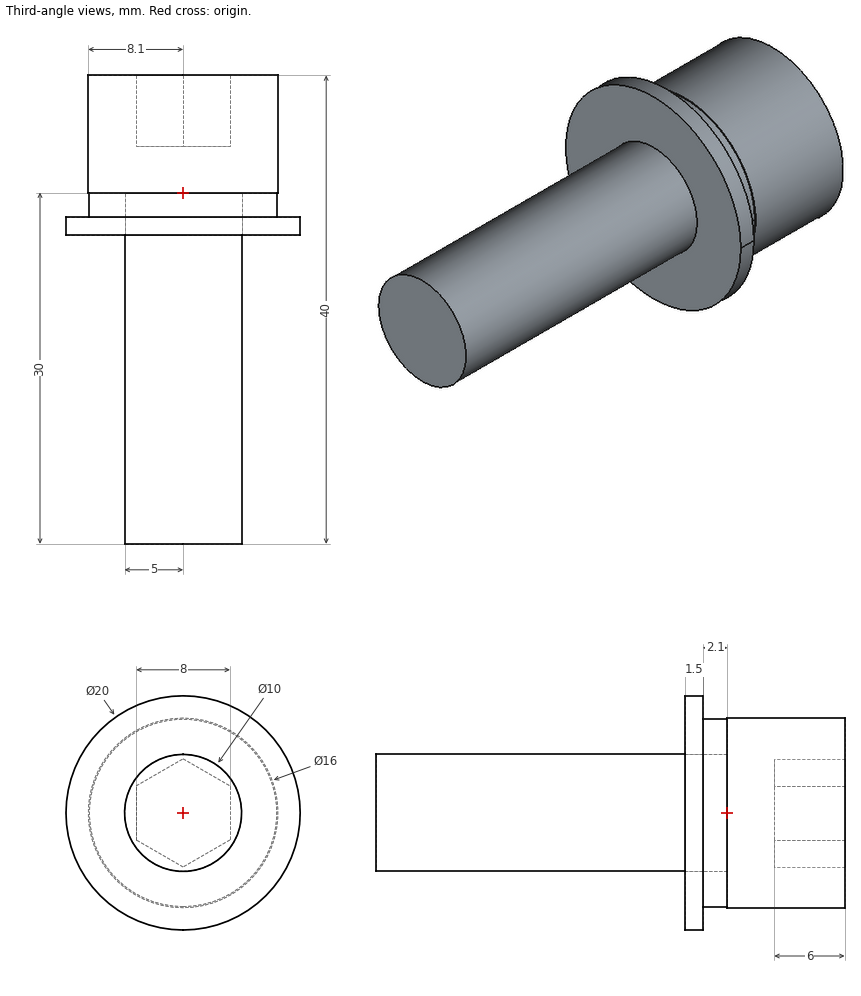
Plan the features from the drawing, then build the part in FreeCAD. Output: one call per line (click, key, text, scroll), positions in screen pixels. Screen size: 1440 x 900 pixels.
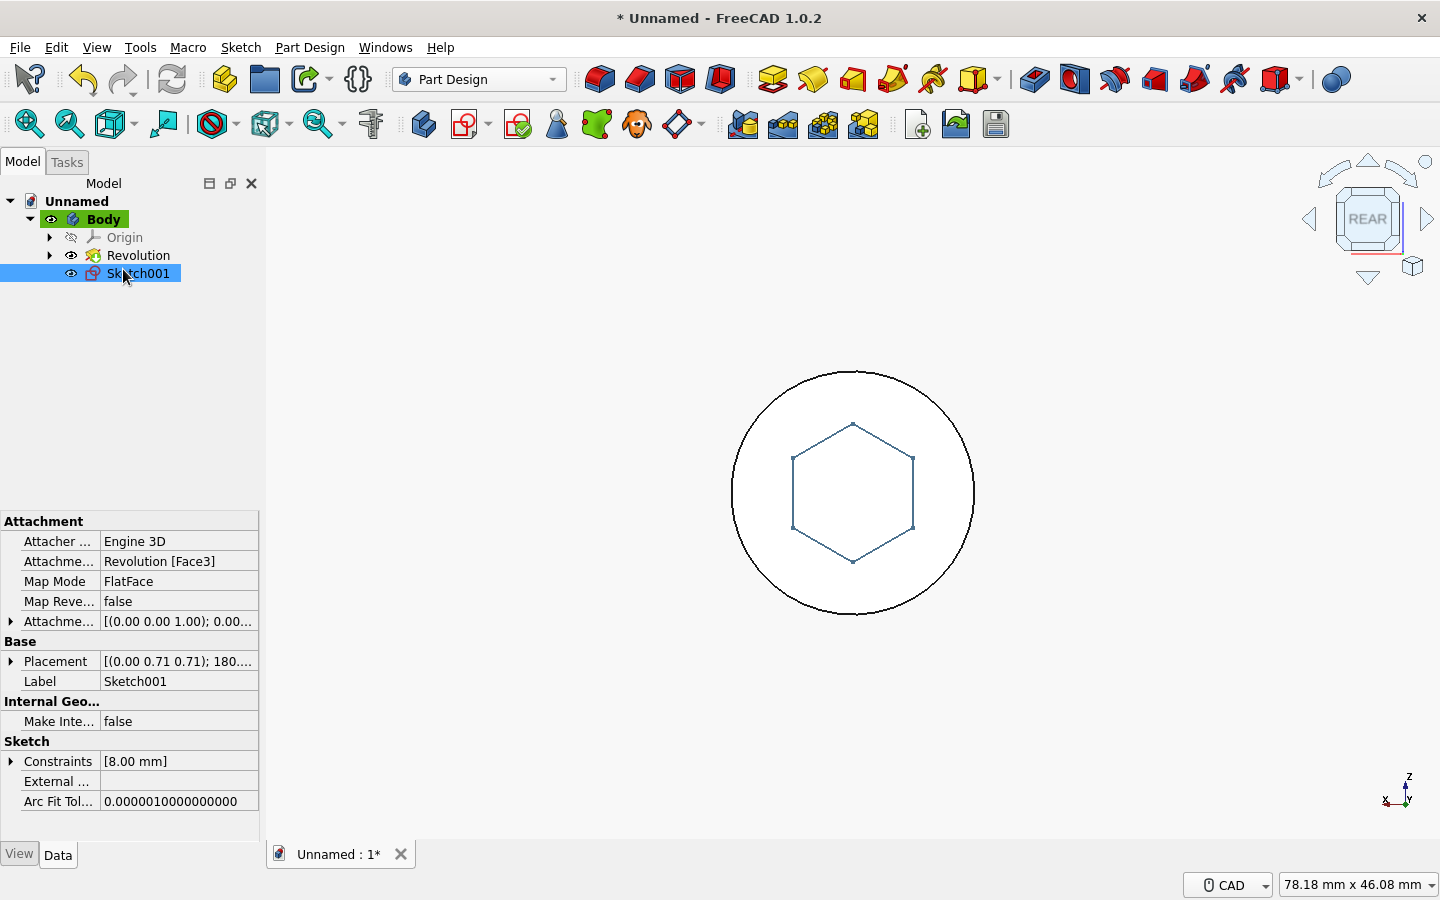
click(1036, 80)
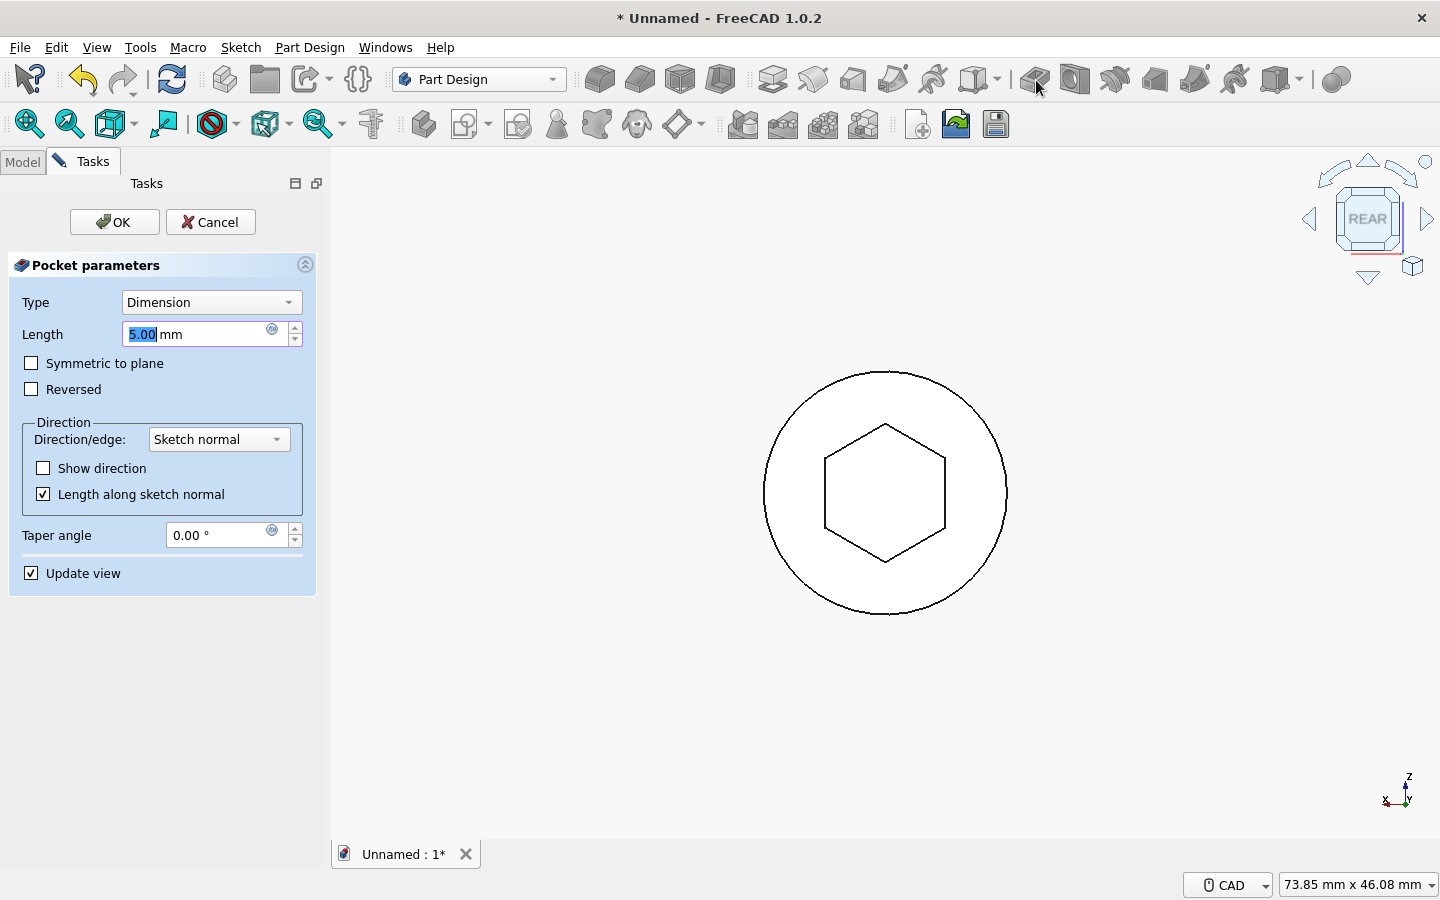
text(6)
key(Tab)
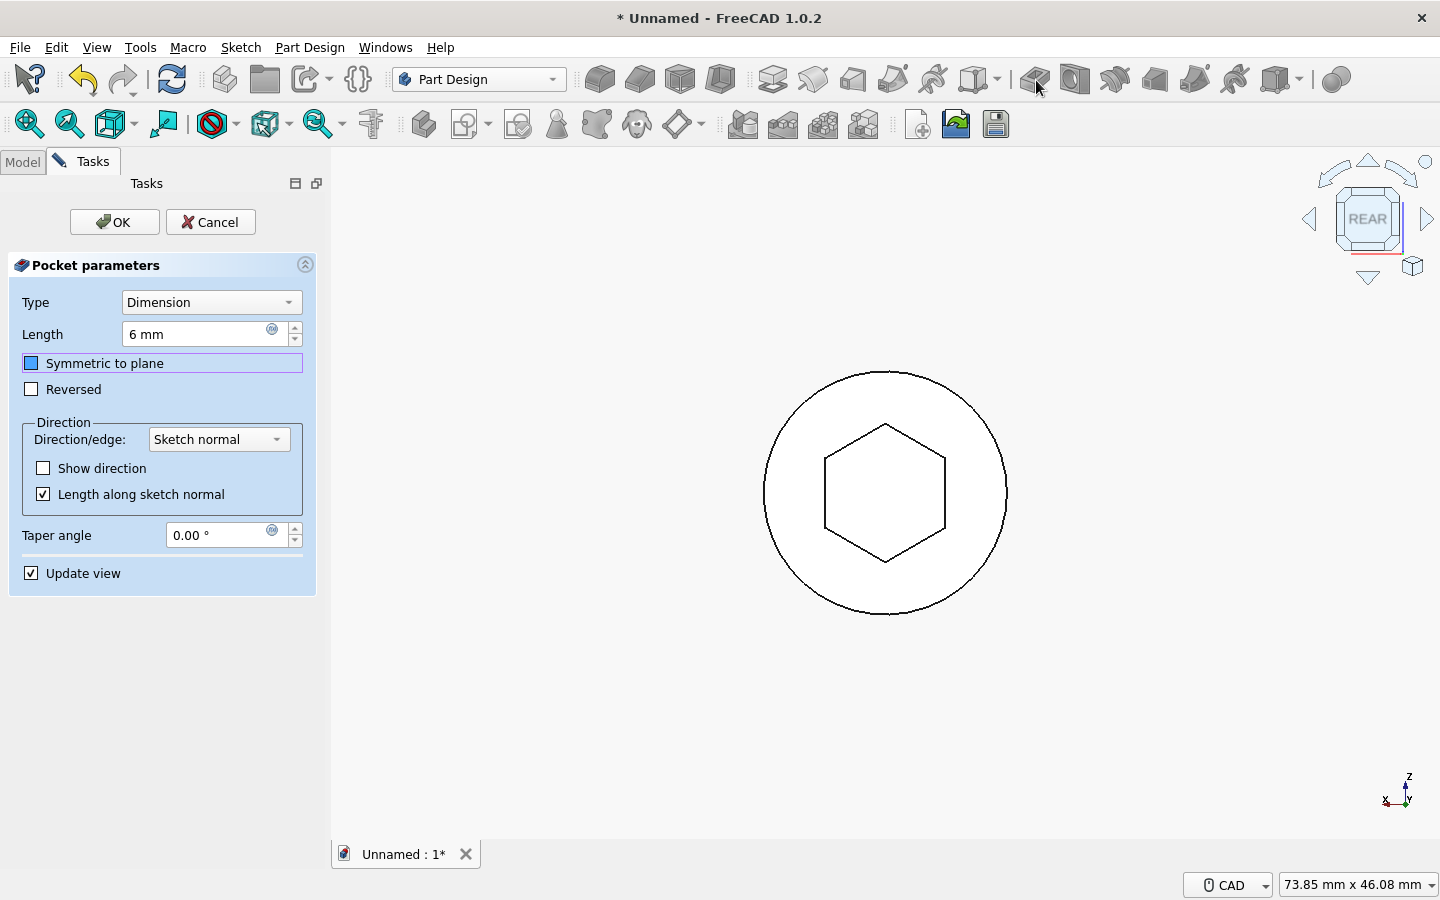
click(115, 222)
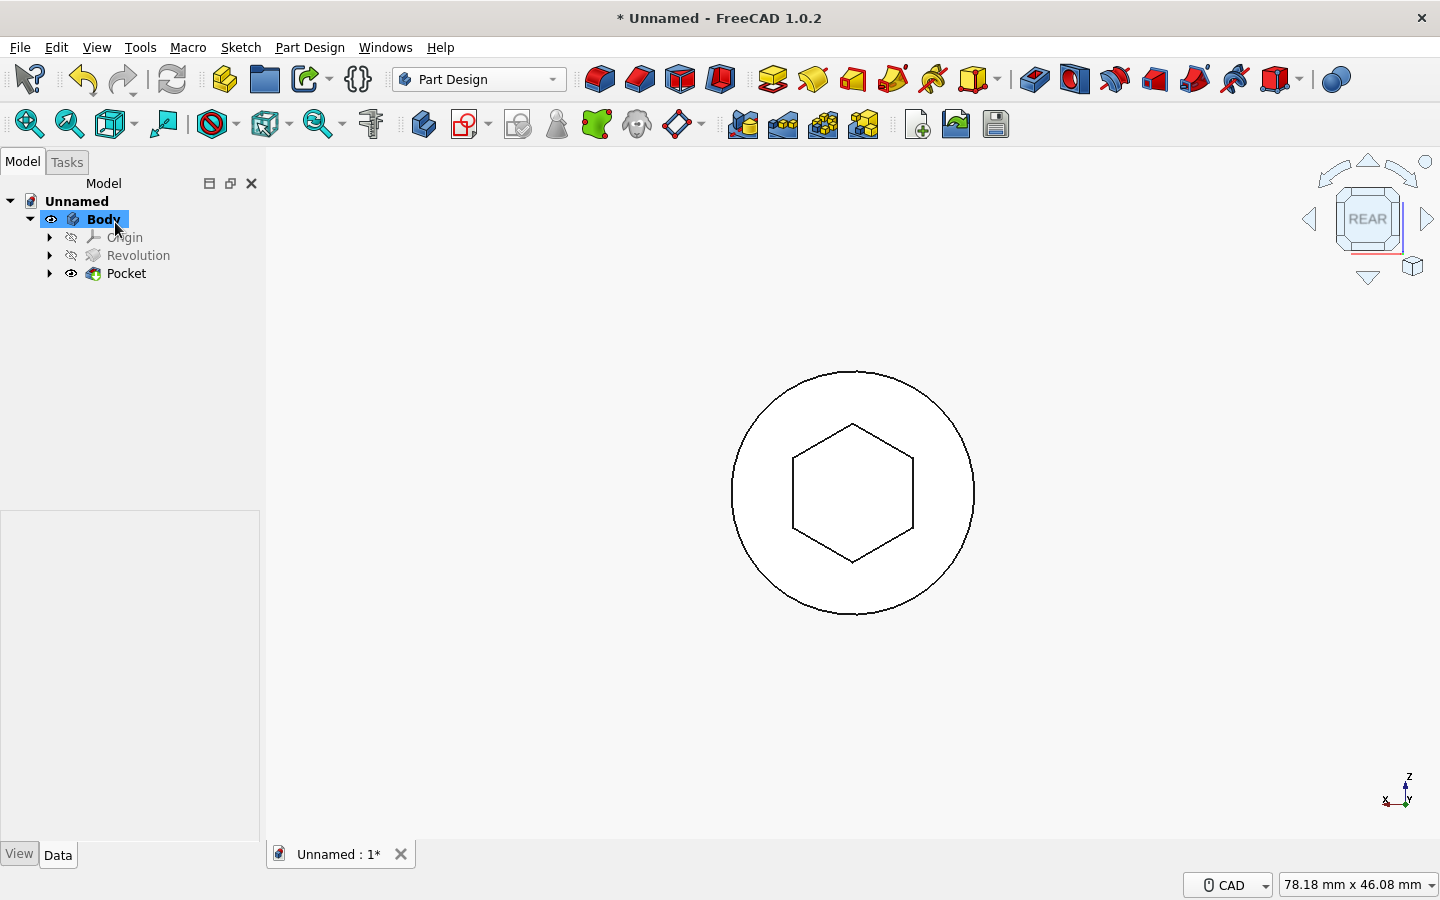
key(v)
key(f)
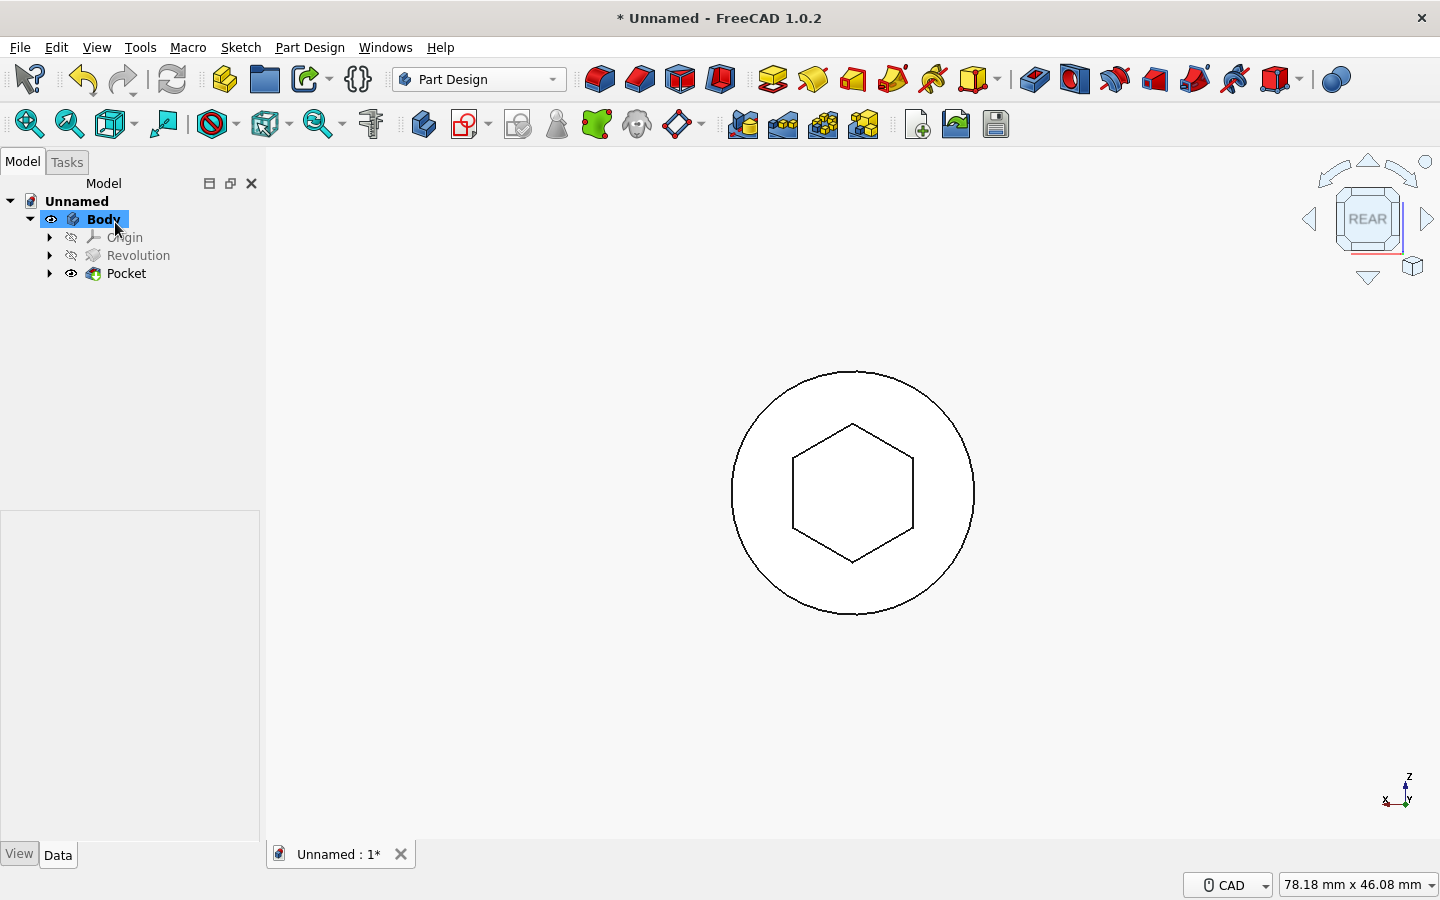
click(424, 124)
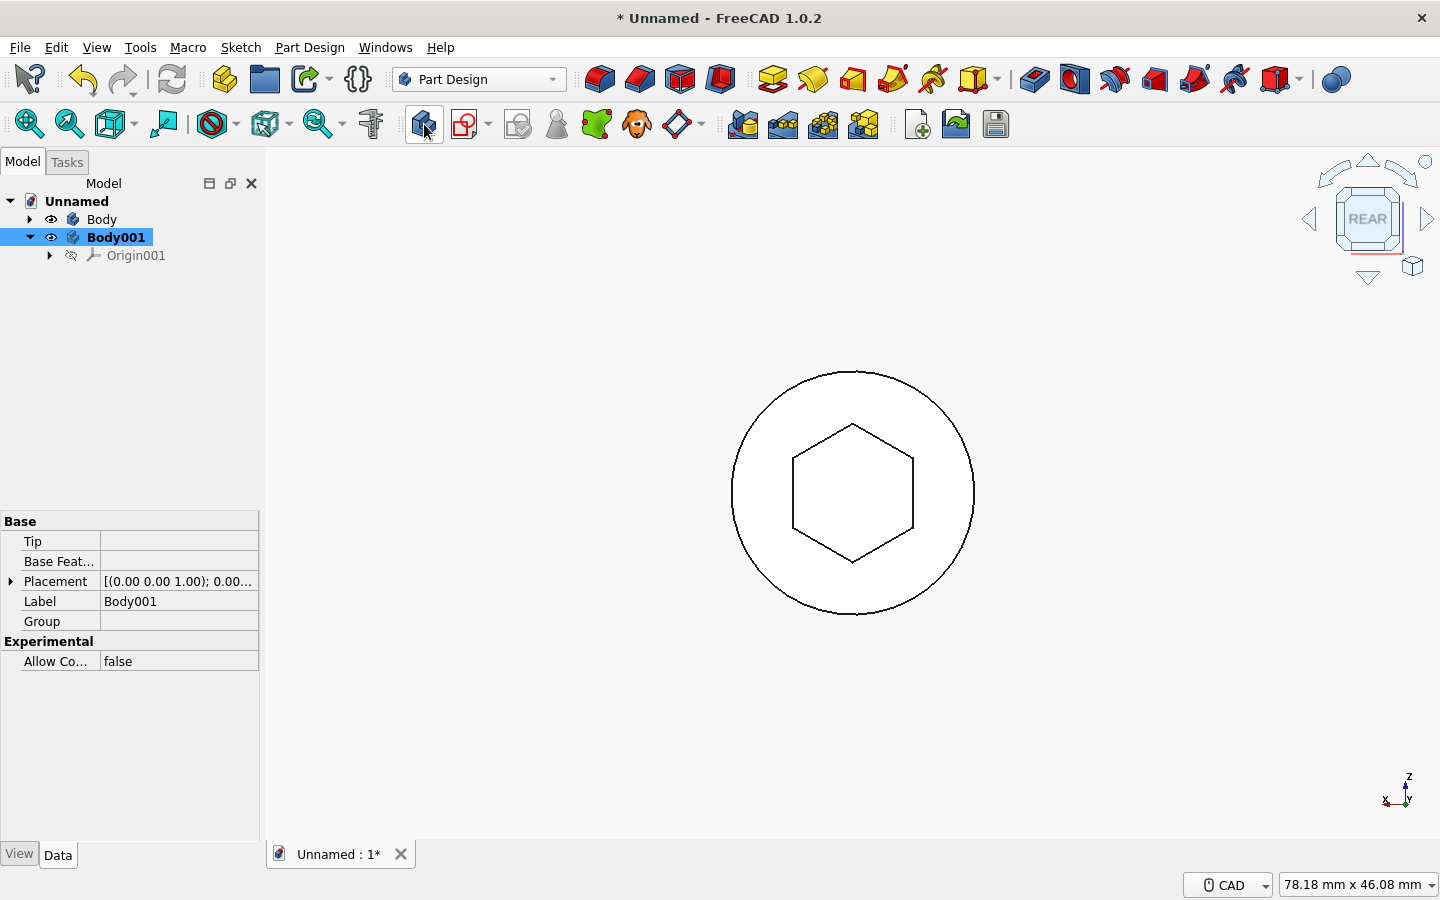
click(306, 799)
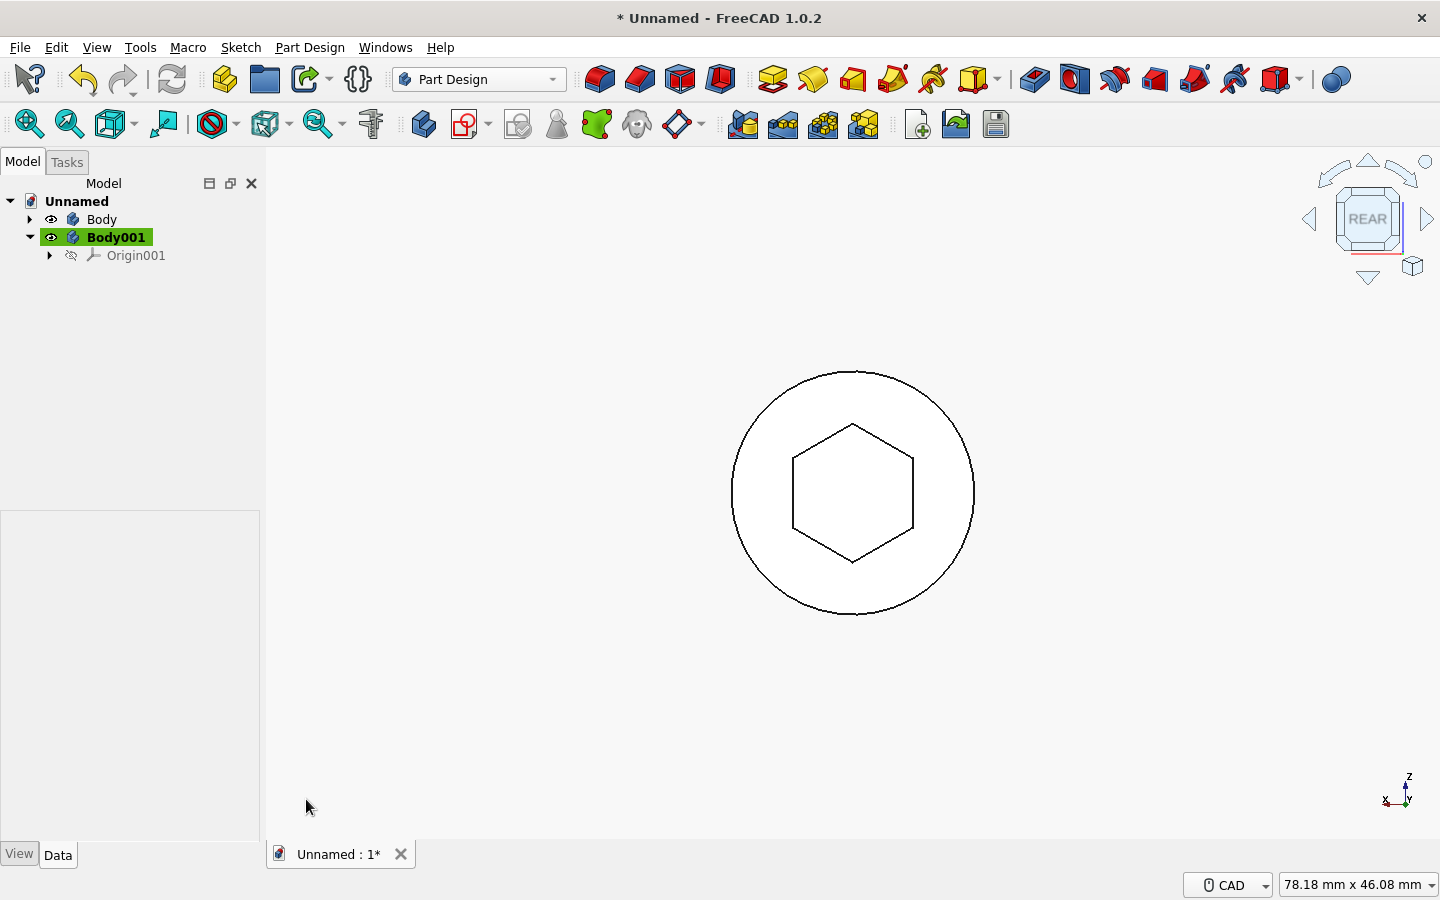
click(464, 124)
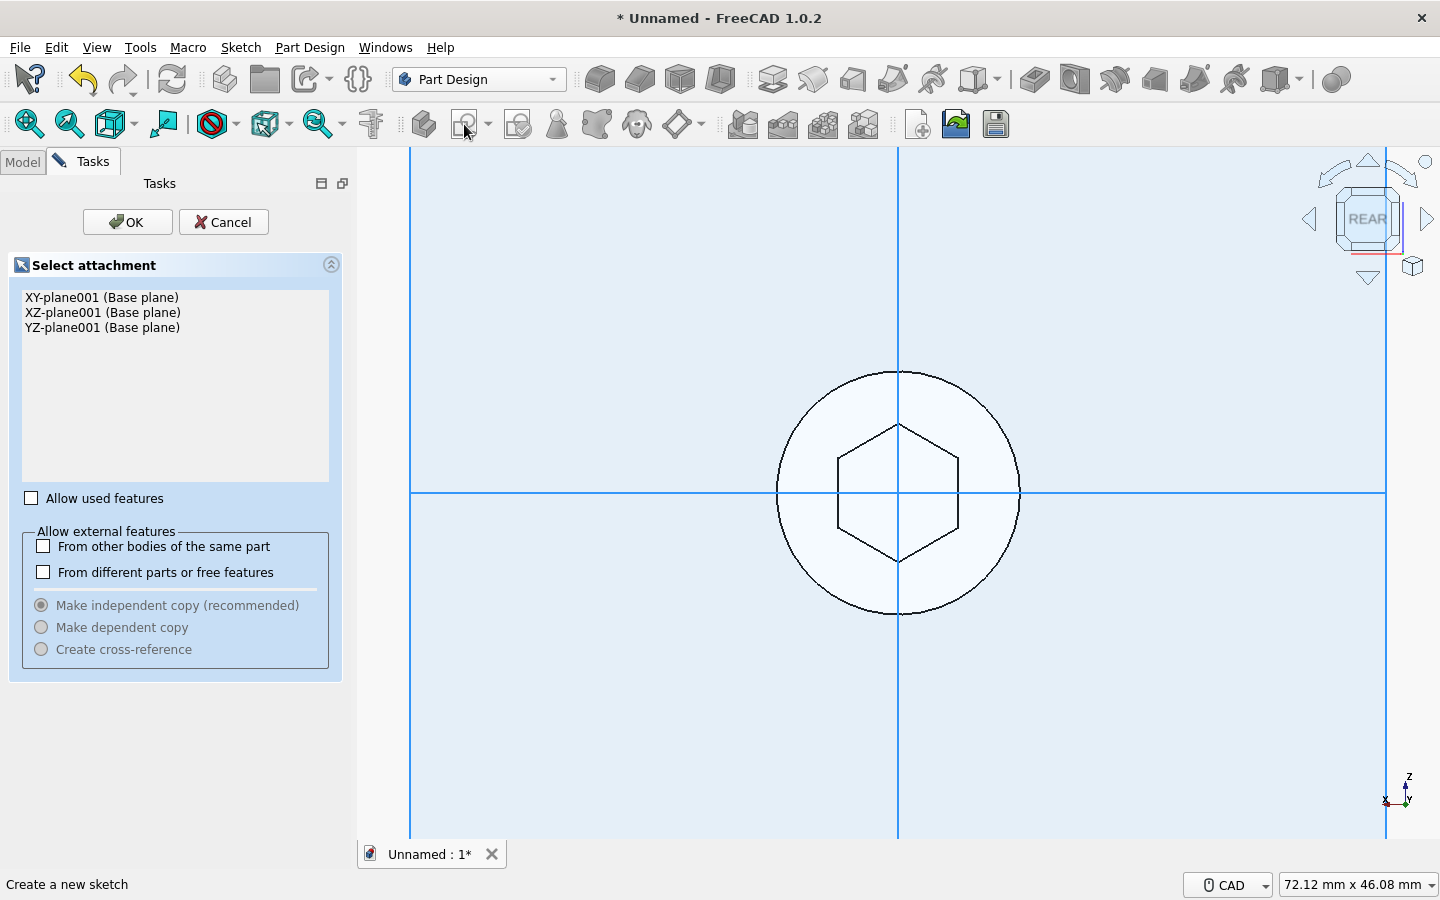
click(82, 312)